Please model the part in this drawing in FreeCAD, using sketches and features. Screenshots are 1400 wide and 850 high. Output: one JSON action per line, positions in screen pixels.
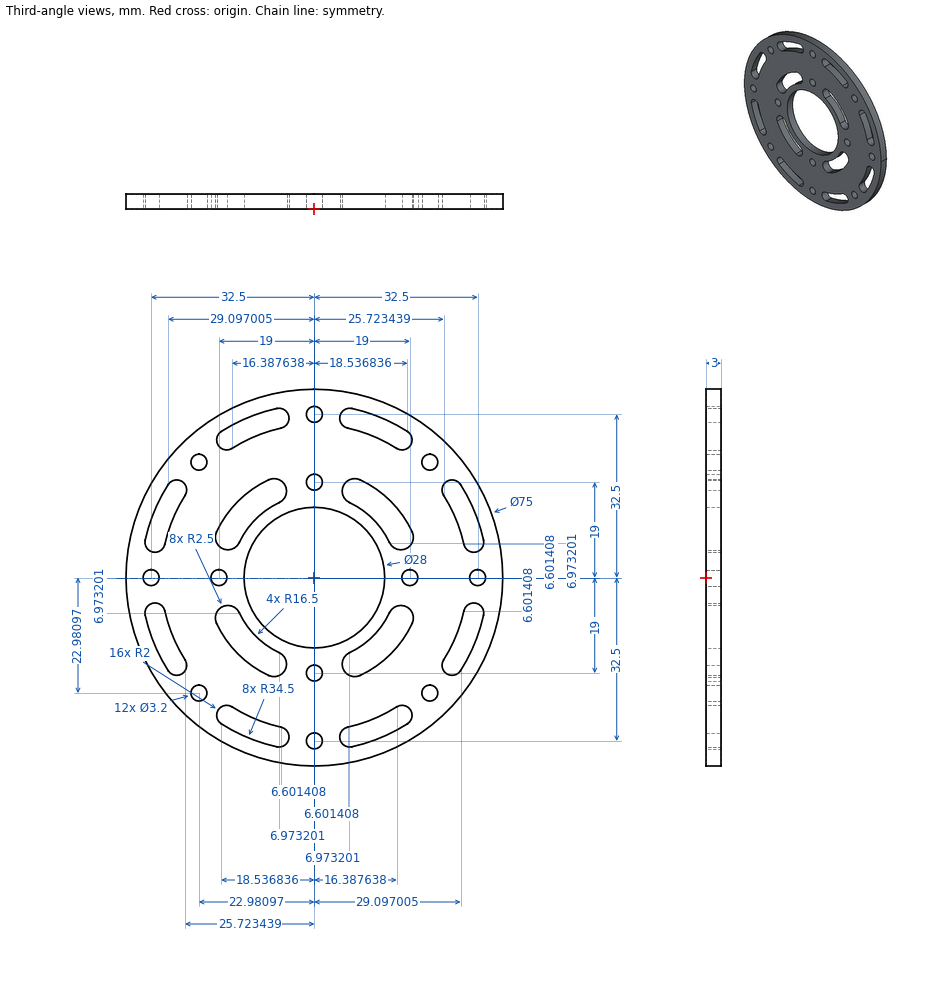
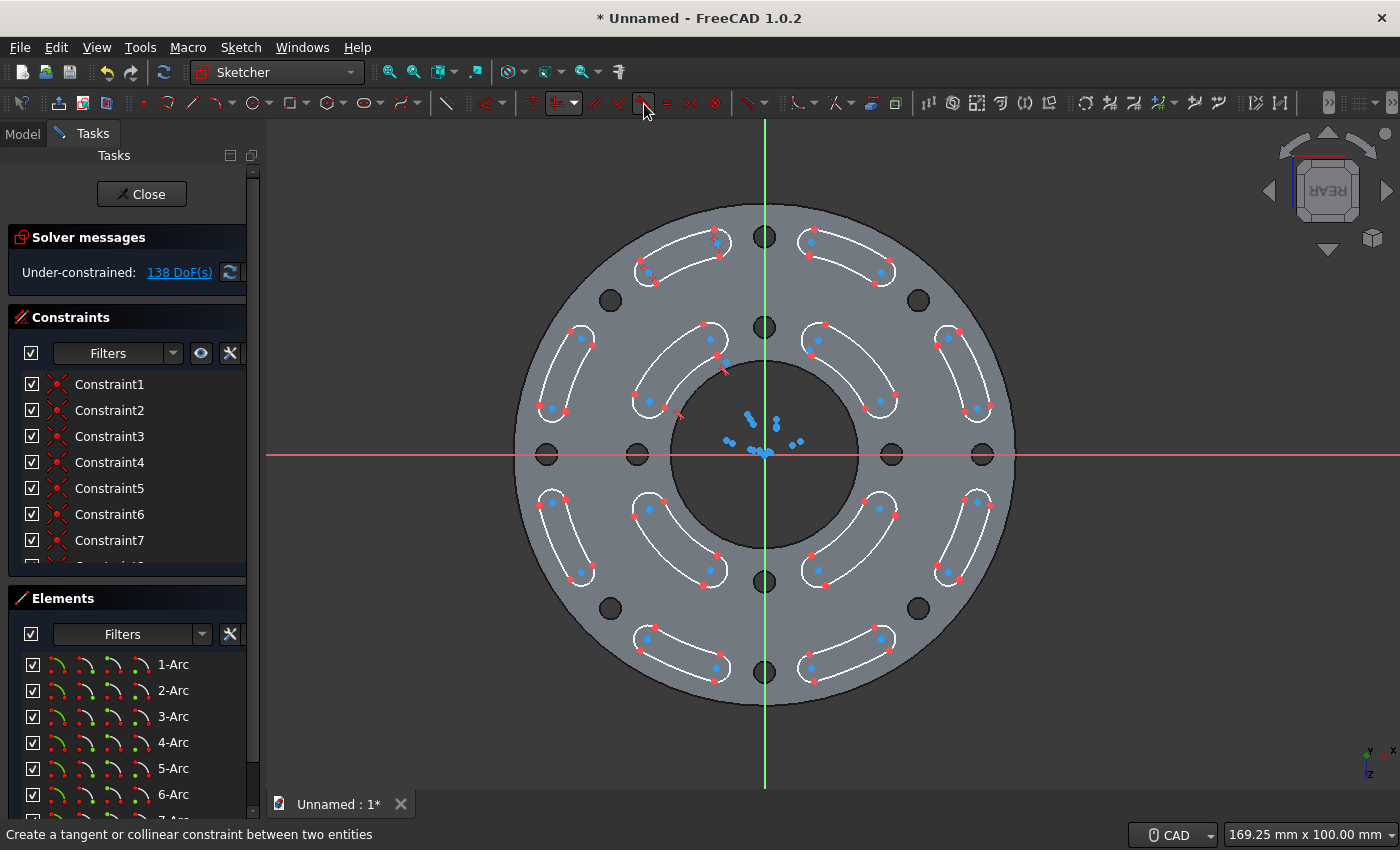
{"action": "left_click", "coordinate": [727, 344]}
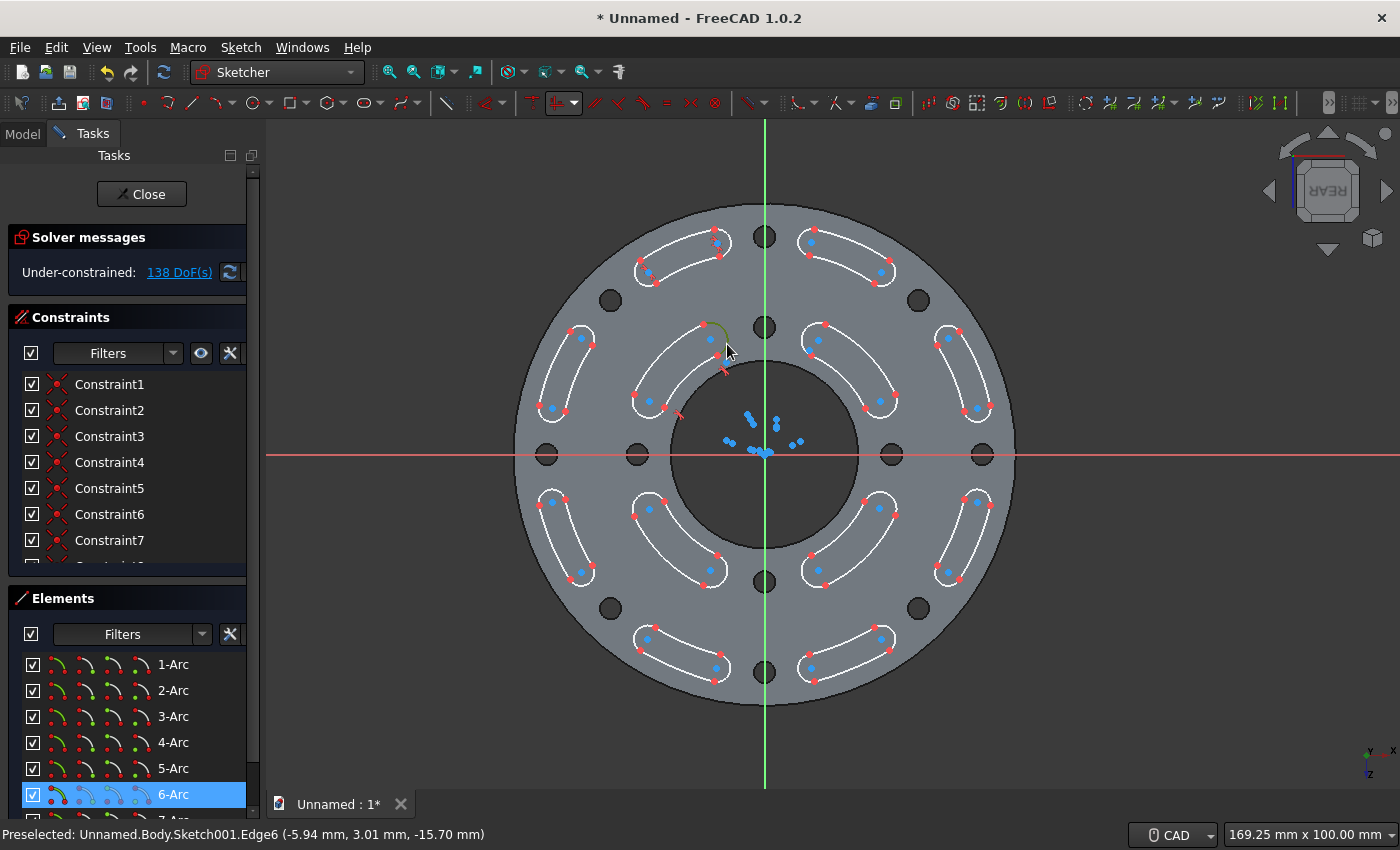
{"action": "left_click", "coordinate": [678, 340]}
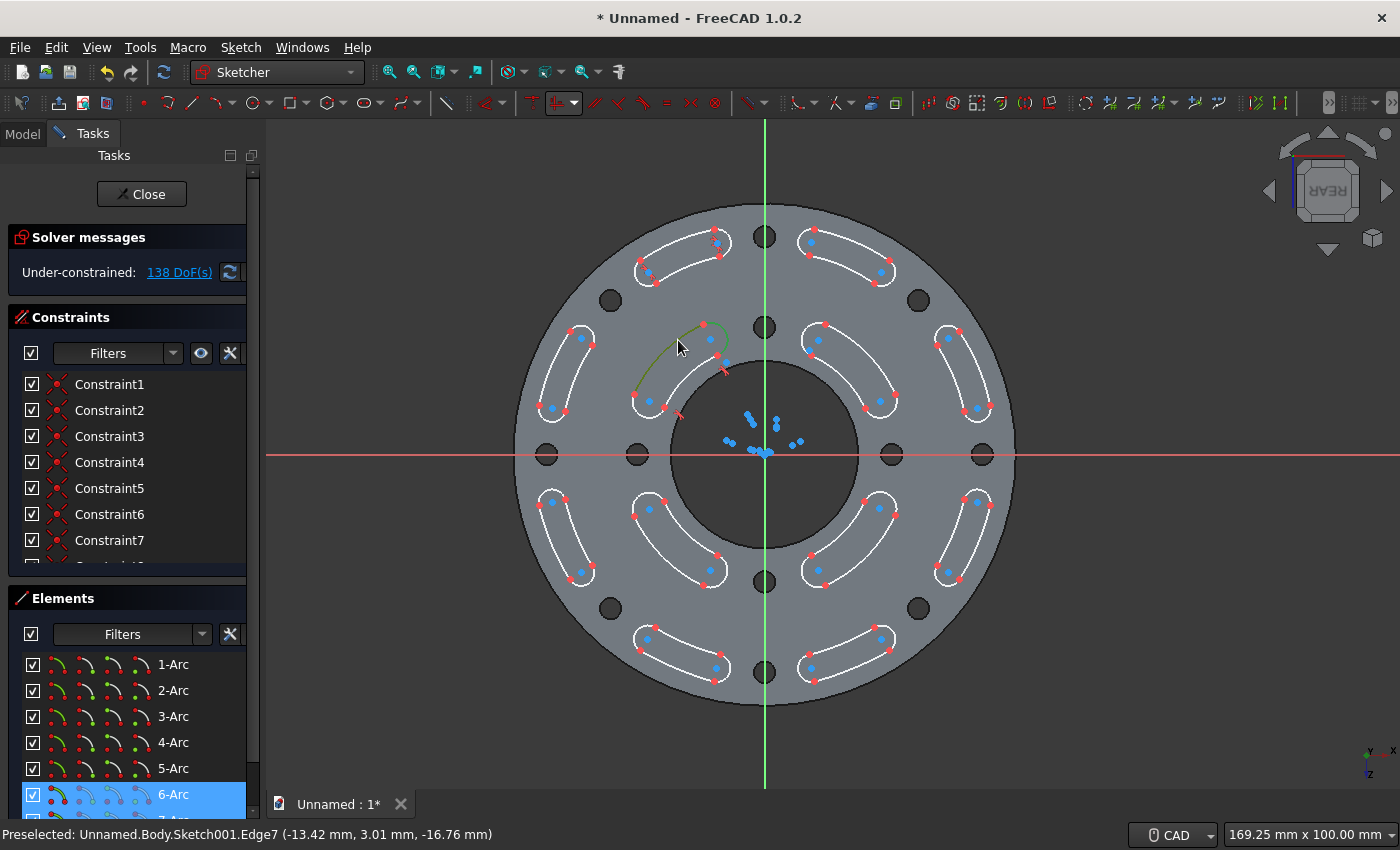
{"action": "left_click", "coordinate": [644, 104]}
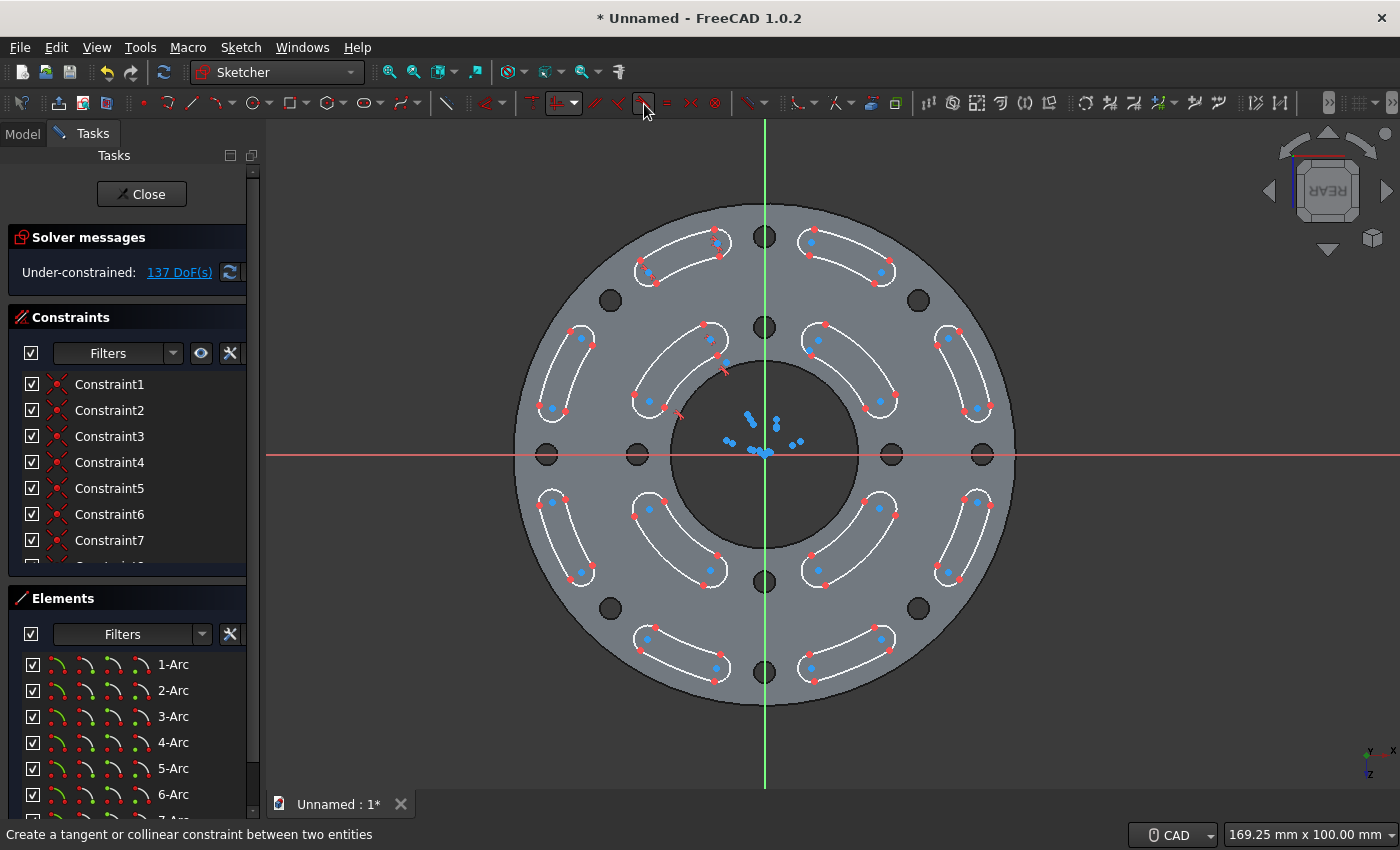
{"action": "left_click", "coordinate": [678, 340]}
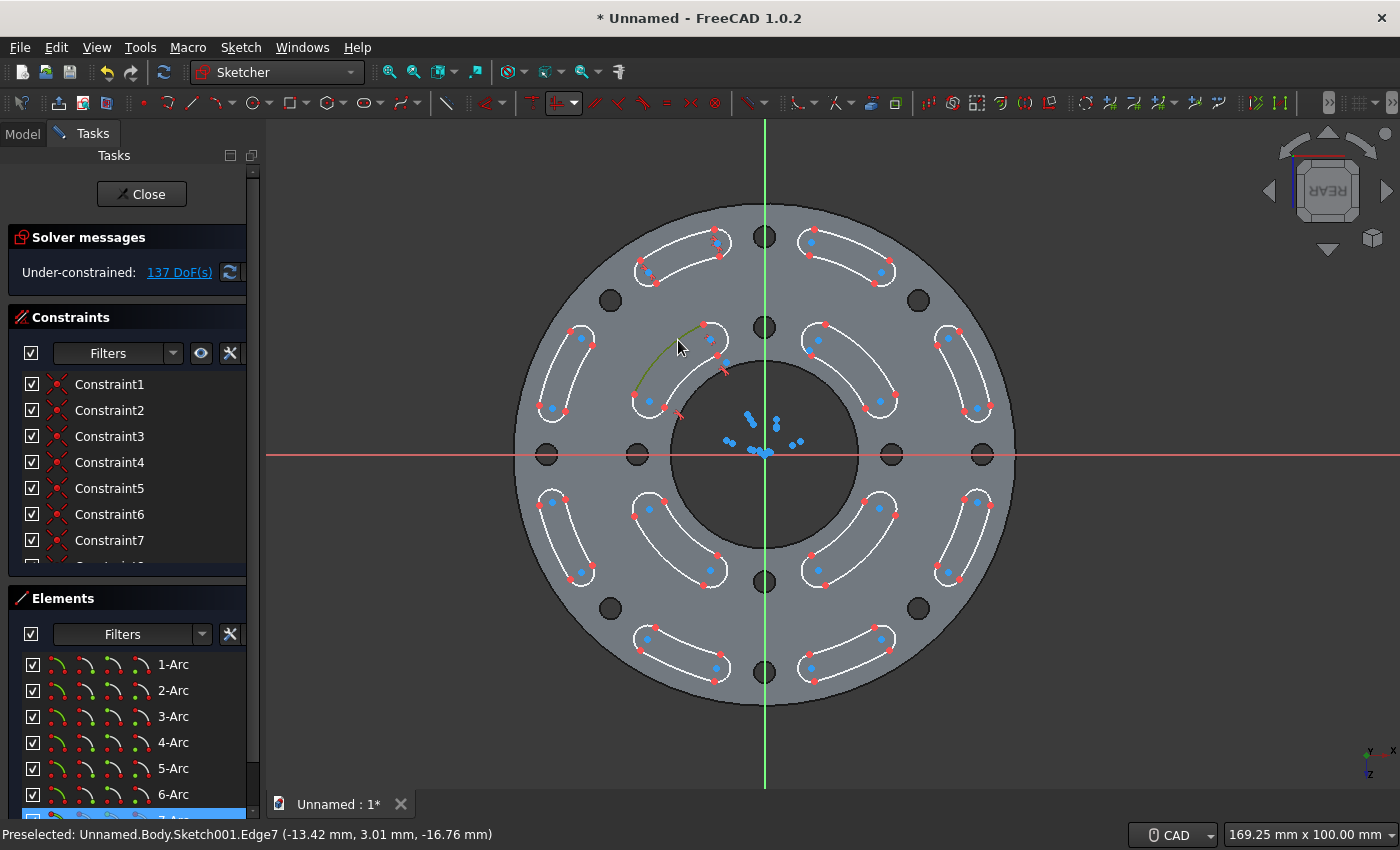
{"action": "left_click", "coordinate": [635, 409]}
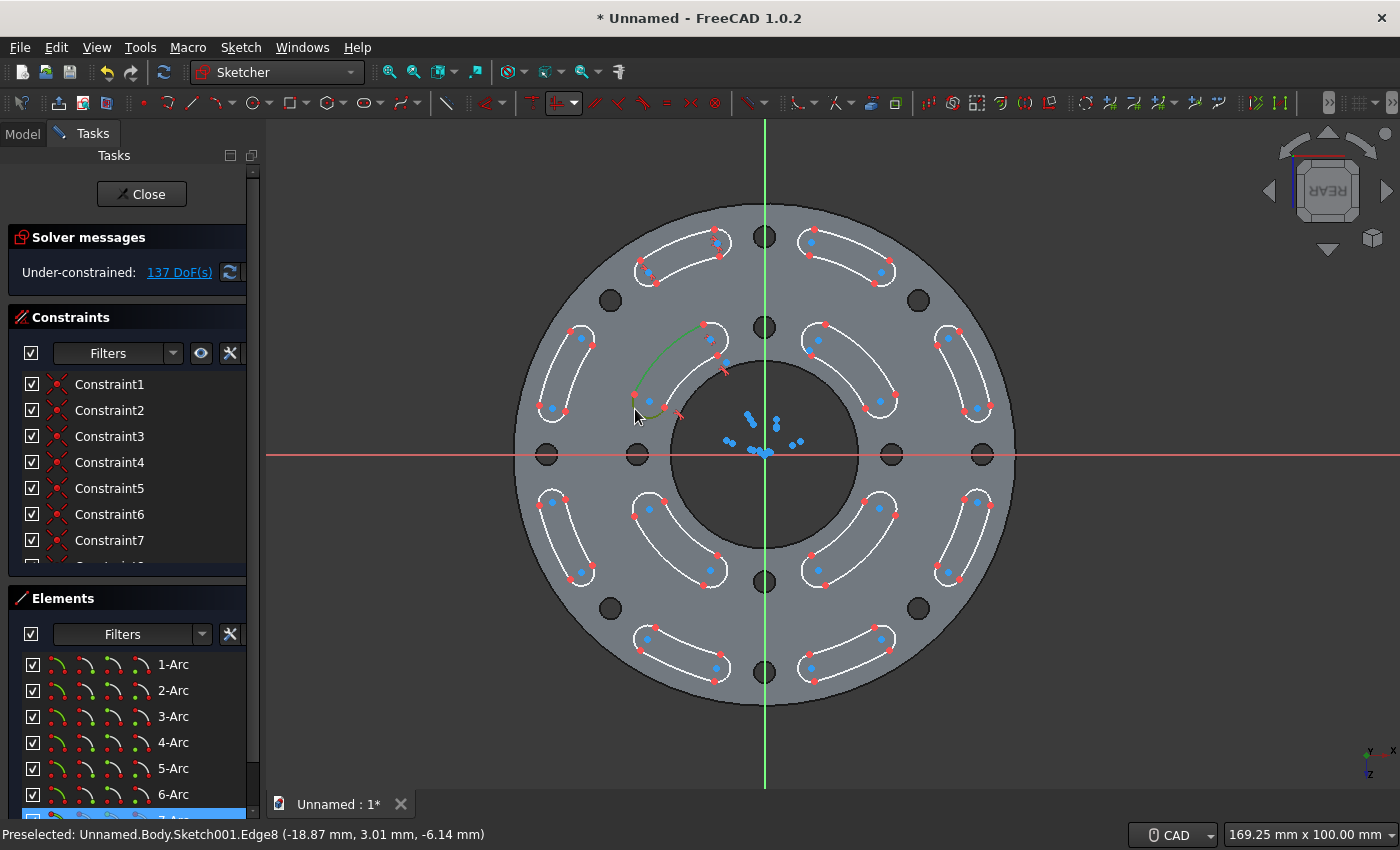
{"action": "left_click", "coordinate": [644, 104]}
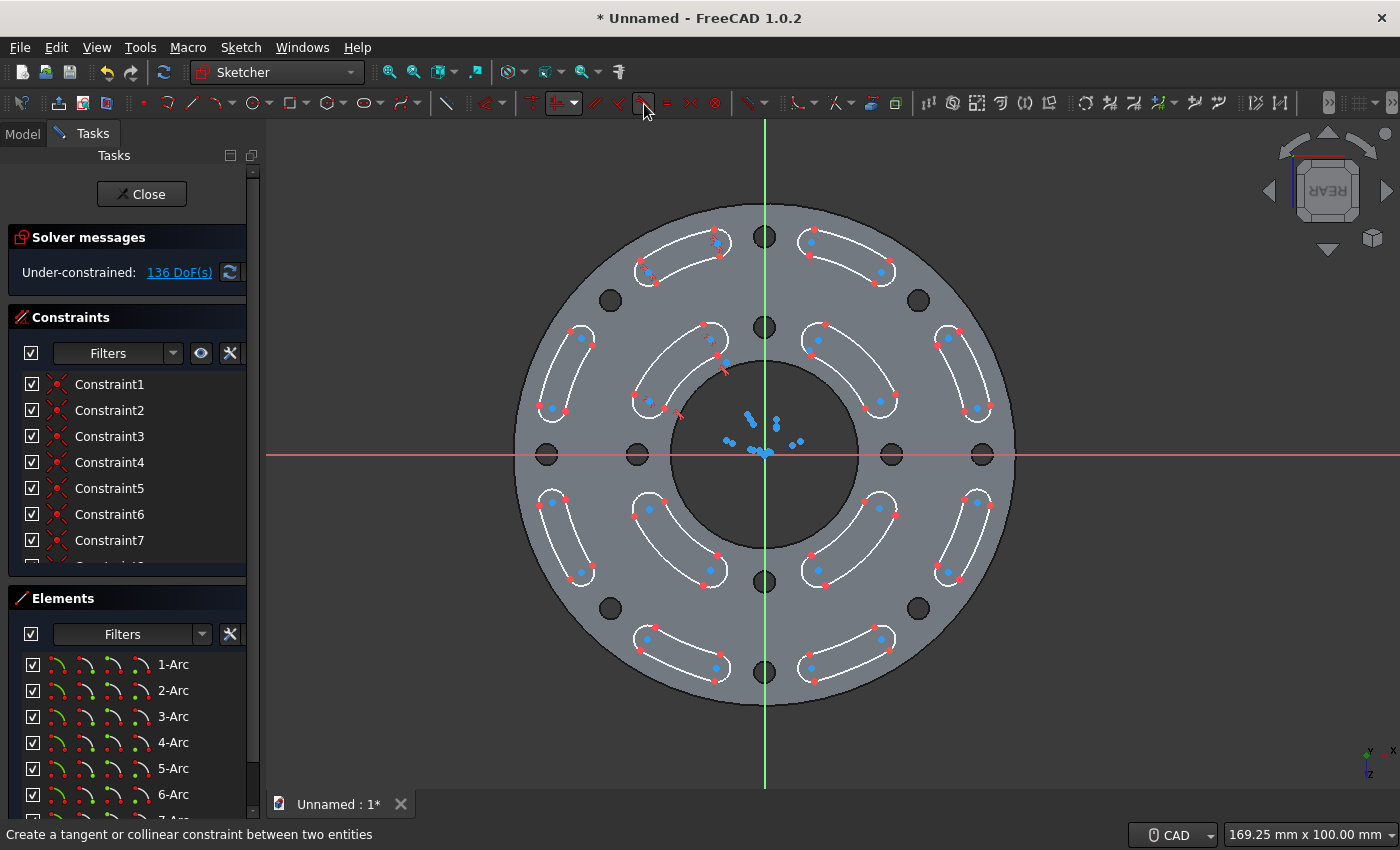
{"action": "left_click", "coordinate": [856, 272]}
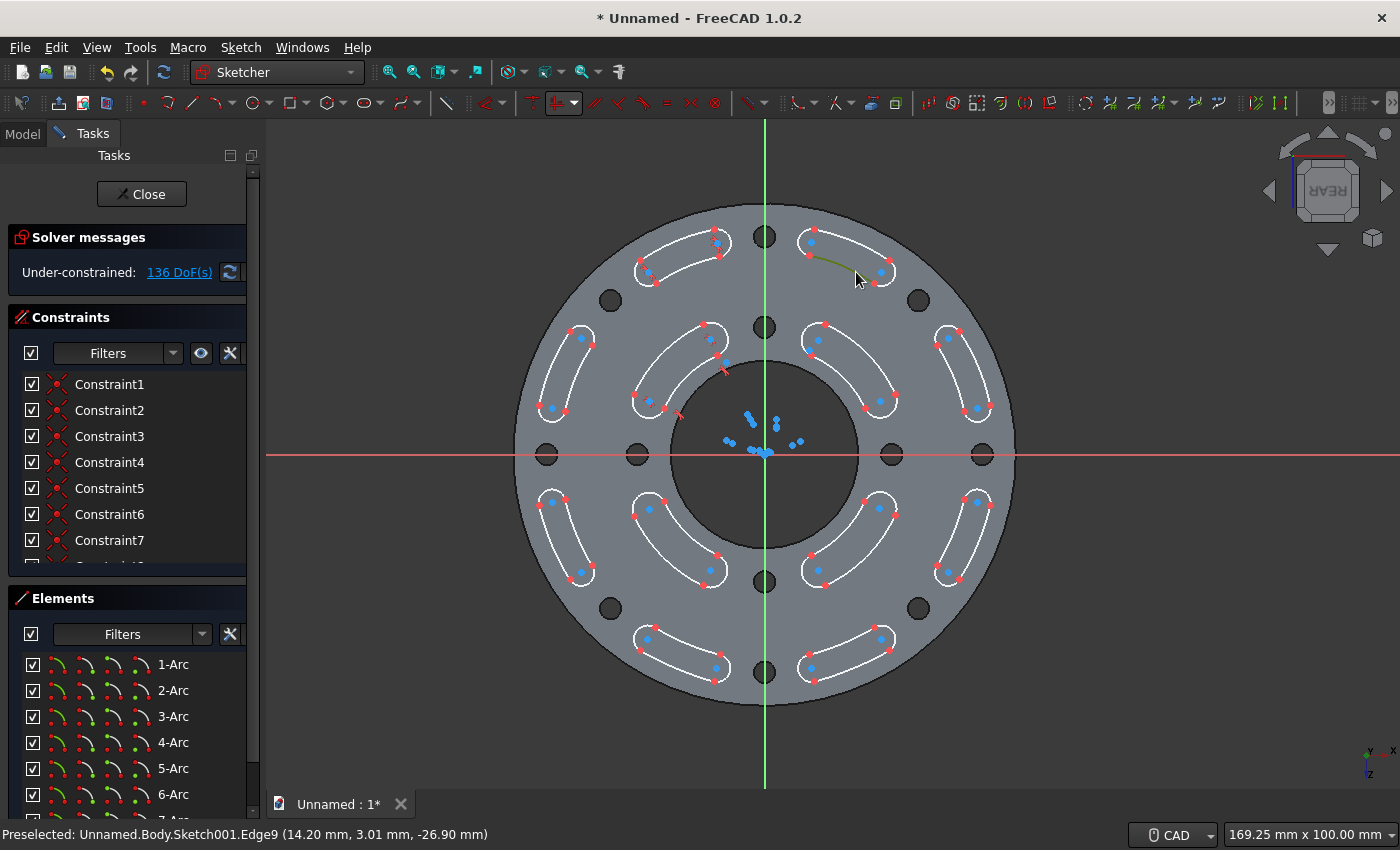
{"action": "left_click", "coordinate": [887, 285]}